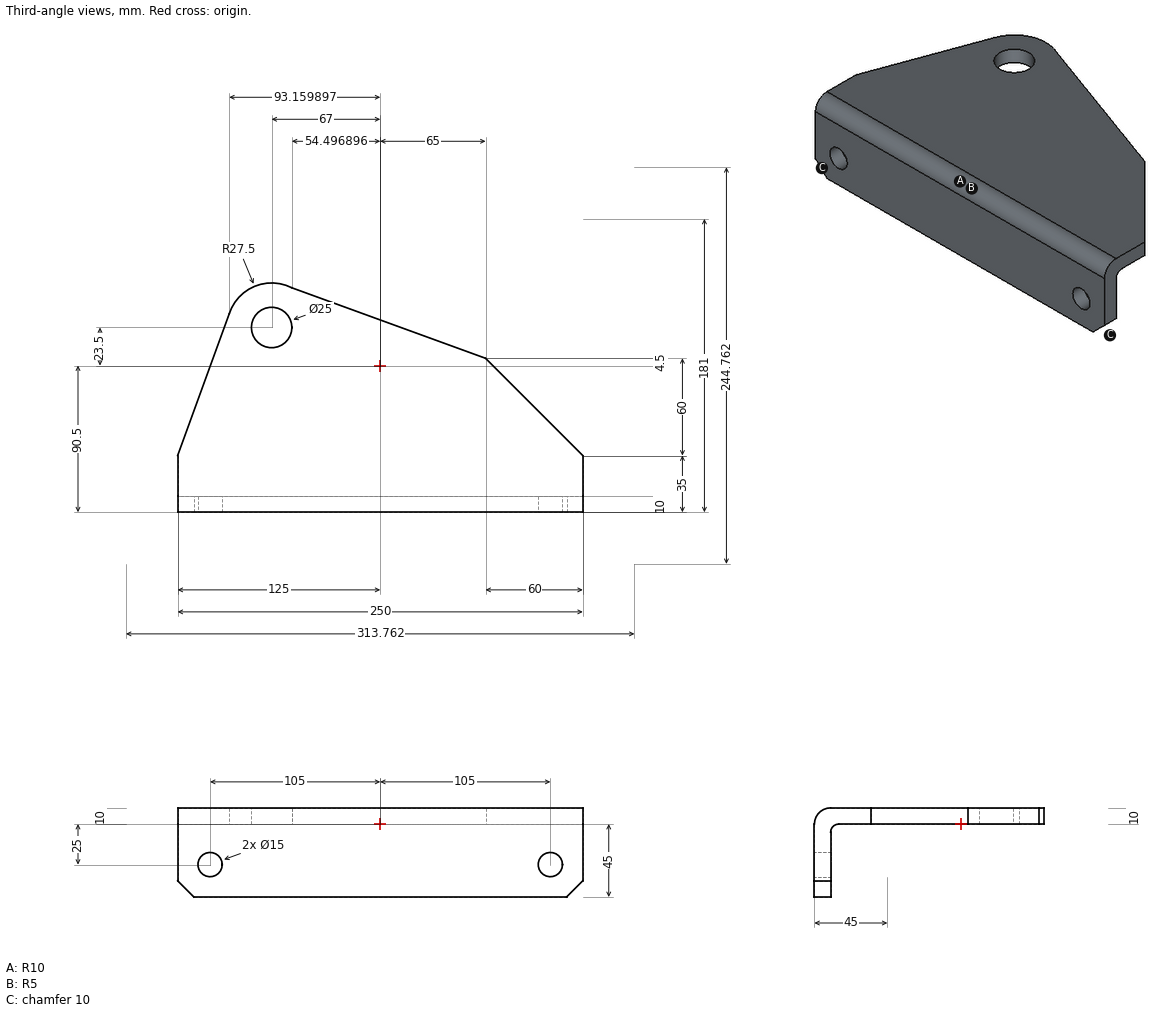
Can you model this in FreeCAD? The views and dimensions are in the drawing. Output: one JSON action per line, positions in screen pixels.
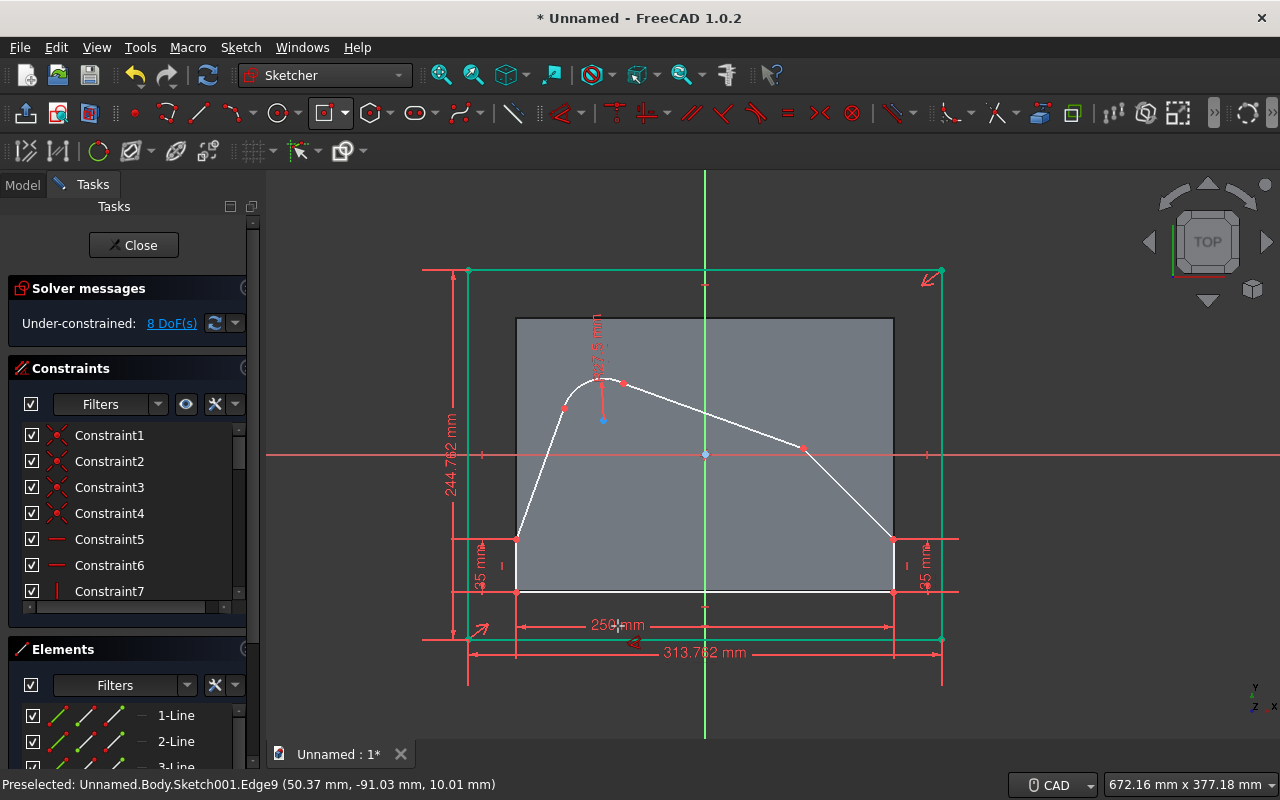
{"action": "left_click", "coordinate": [803, 449]}
{"action": "left_click", "coordinate": [754, 415]}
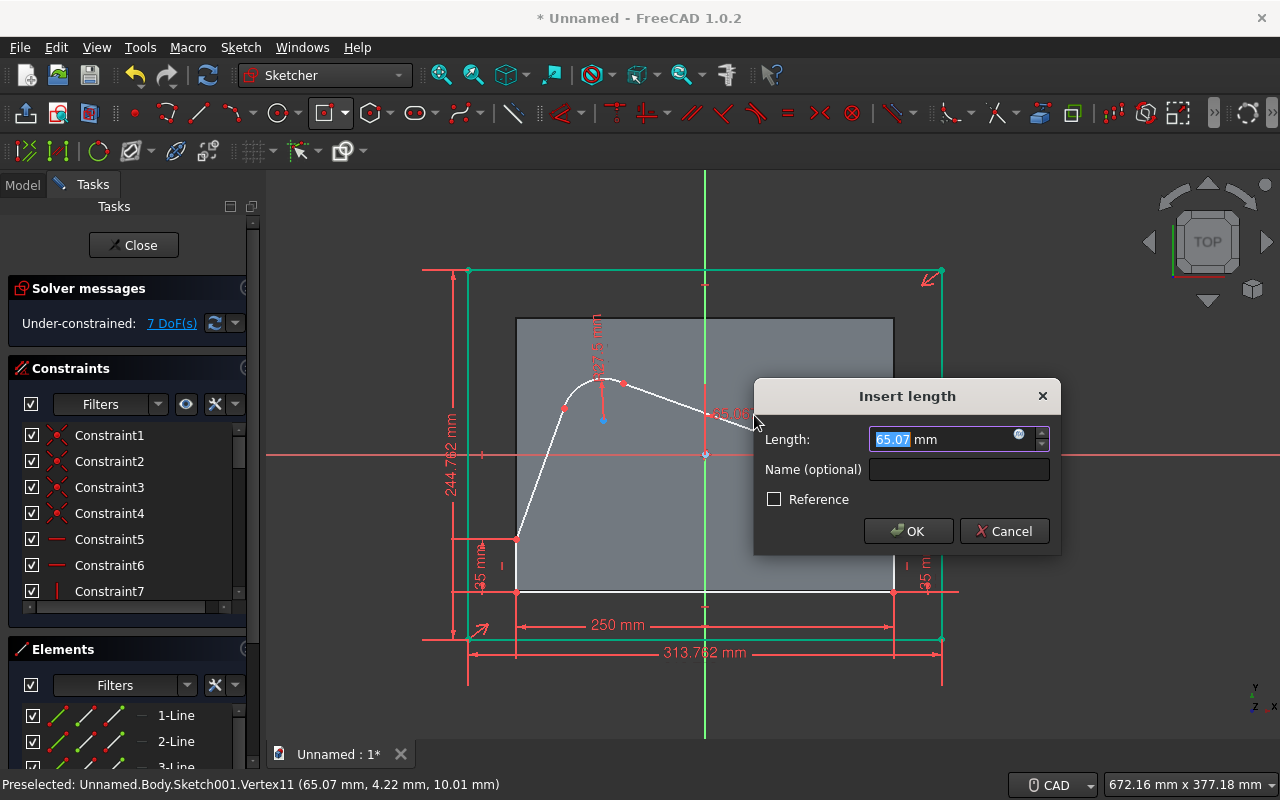
{"action": "type", "text": "65"}
{"action": "key", "text": "Return"}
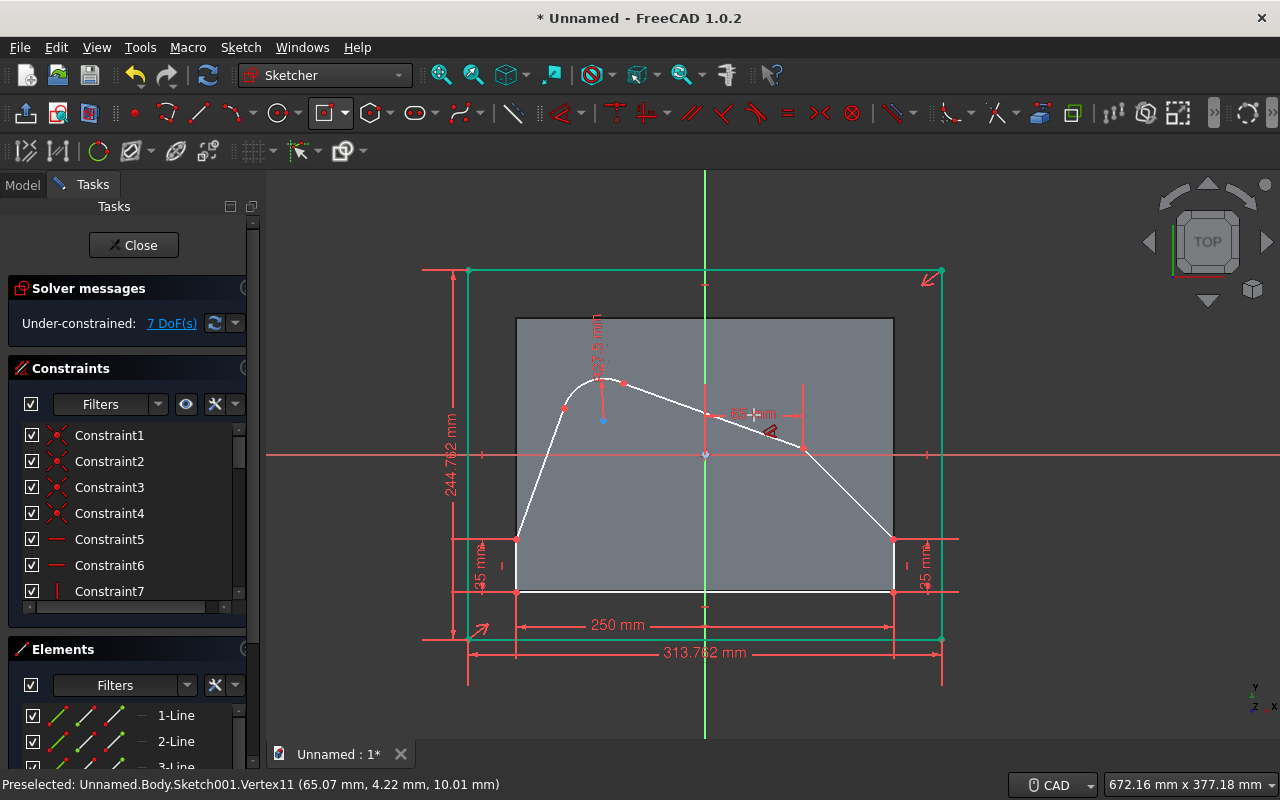
{"action": "left_click", "coordinate": [830, 476]}
{"action": "left_click", "coordinate": [848, 573]}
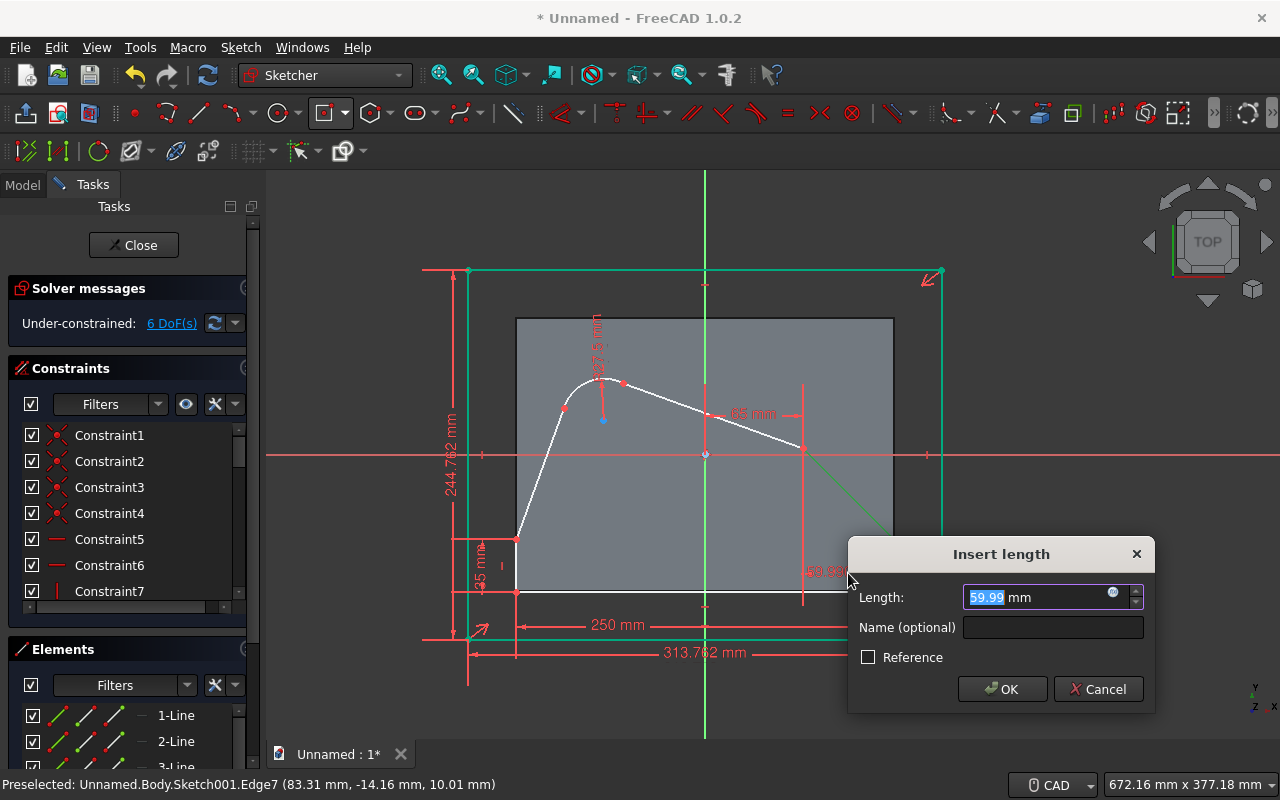
{"action": "type", "text": "60"}
{"action": "key", "text": "Return"}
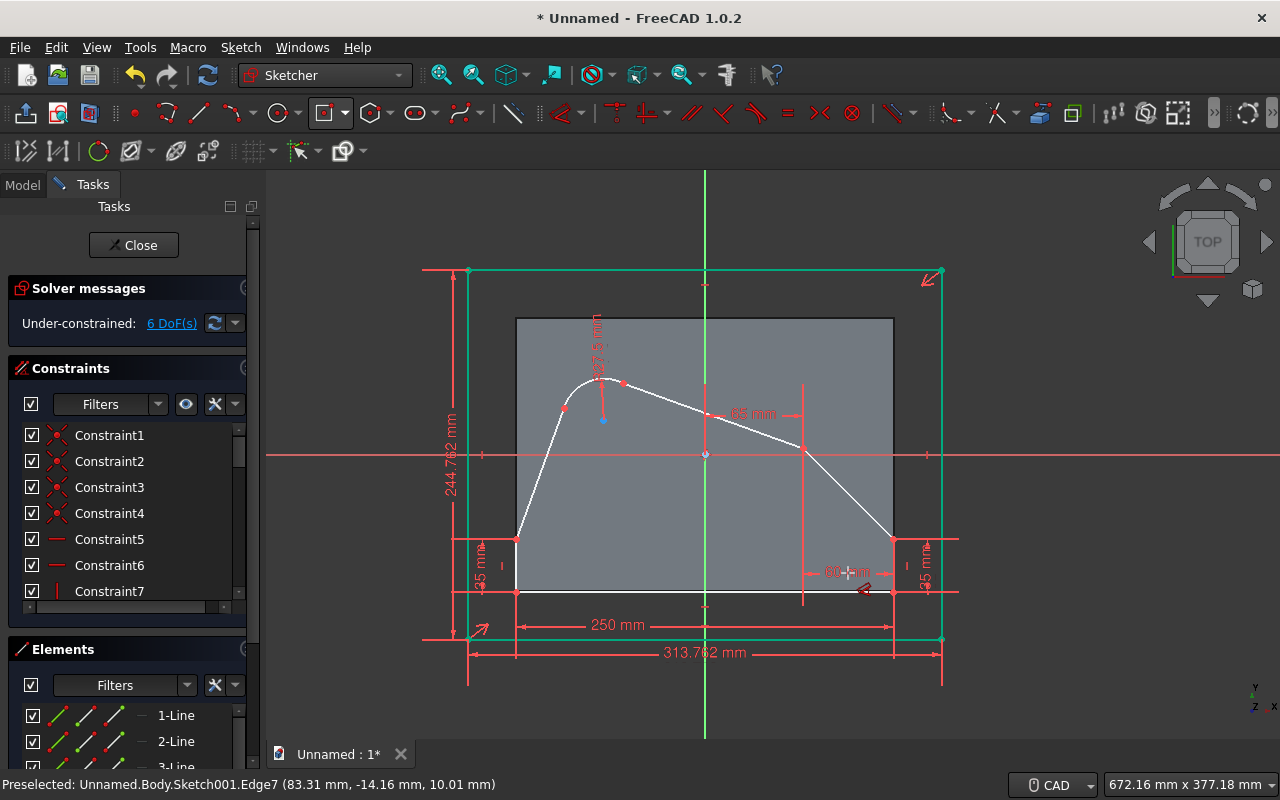
{"action": "left_click", "coordinate": [830, 476]}
{"action": "left_click", "coordinate": [928, 494]}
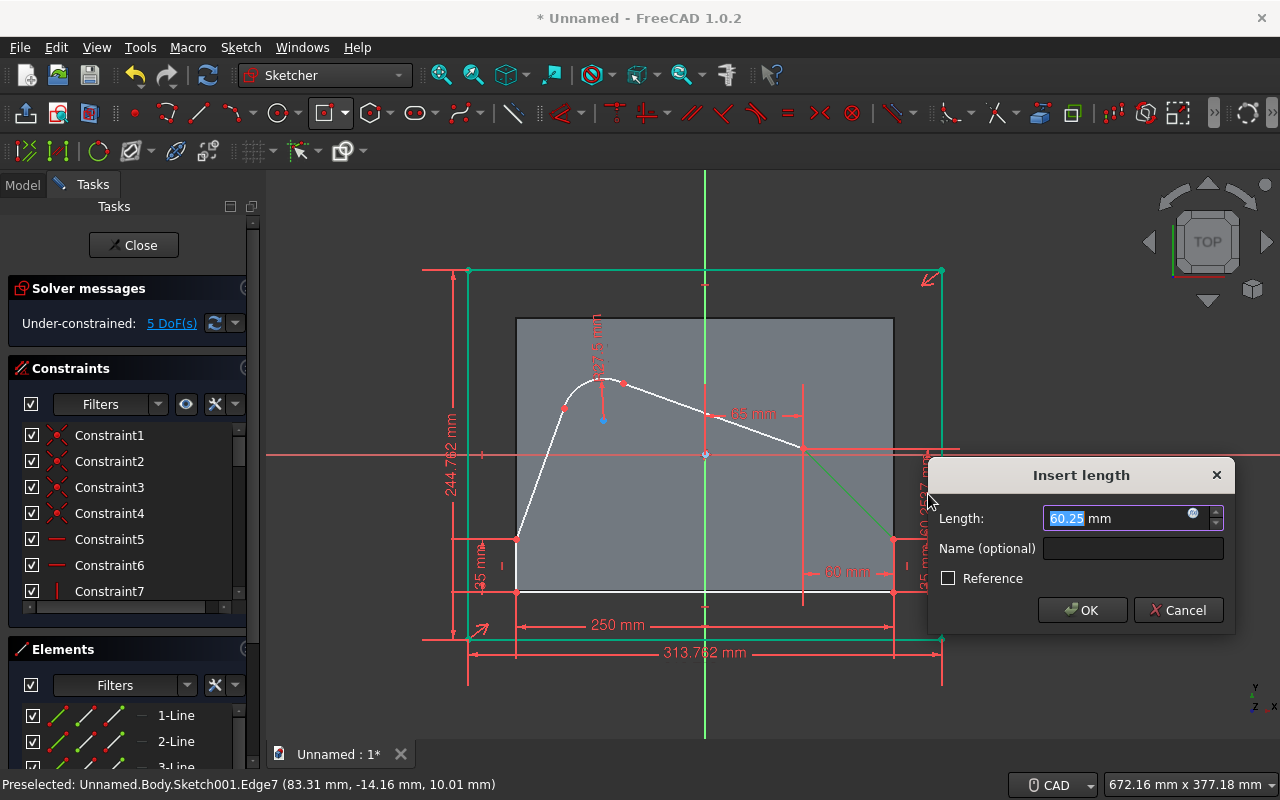
{"action": "type", "text": "60"}
{"action": "key", "text": "Return"}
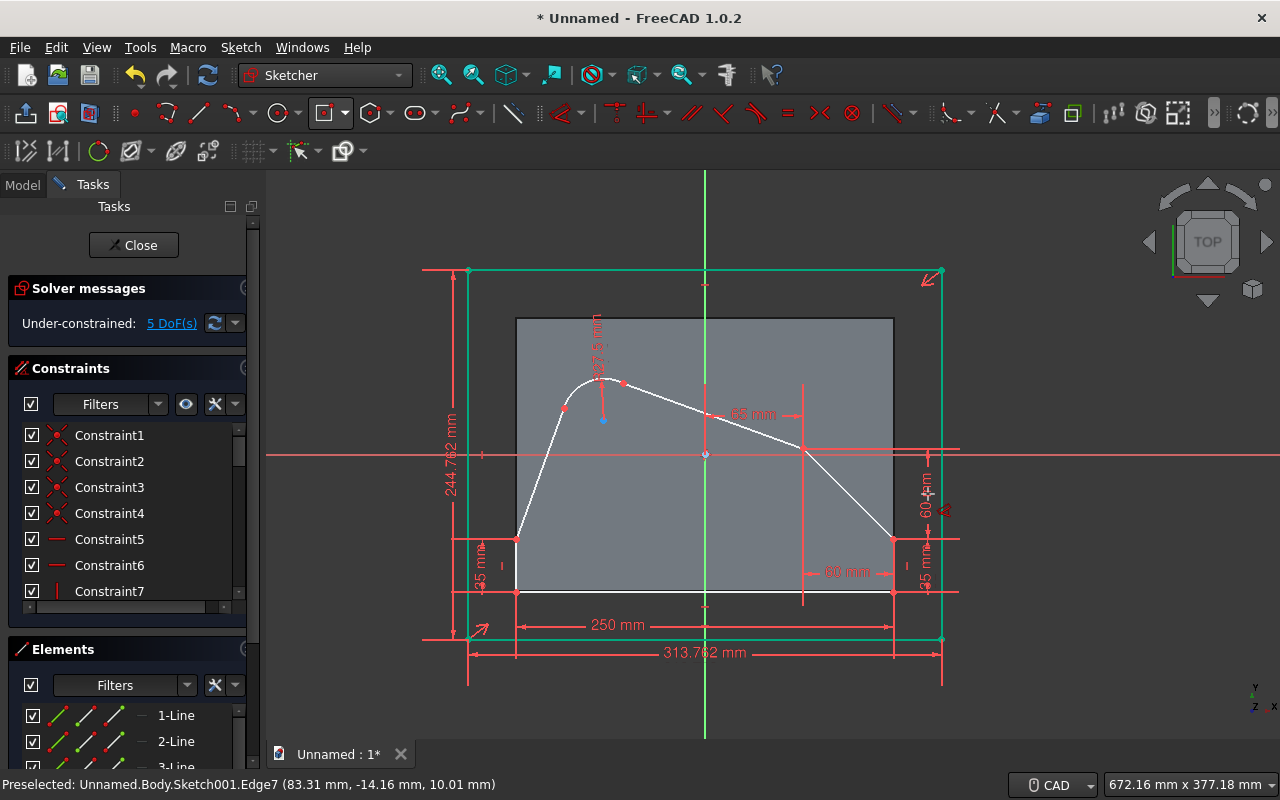
{"action": "left_click", "coordinate": [604, 420]}
{"action": "left_click", "coordinate": [678, 386]}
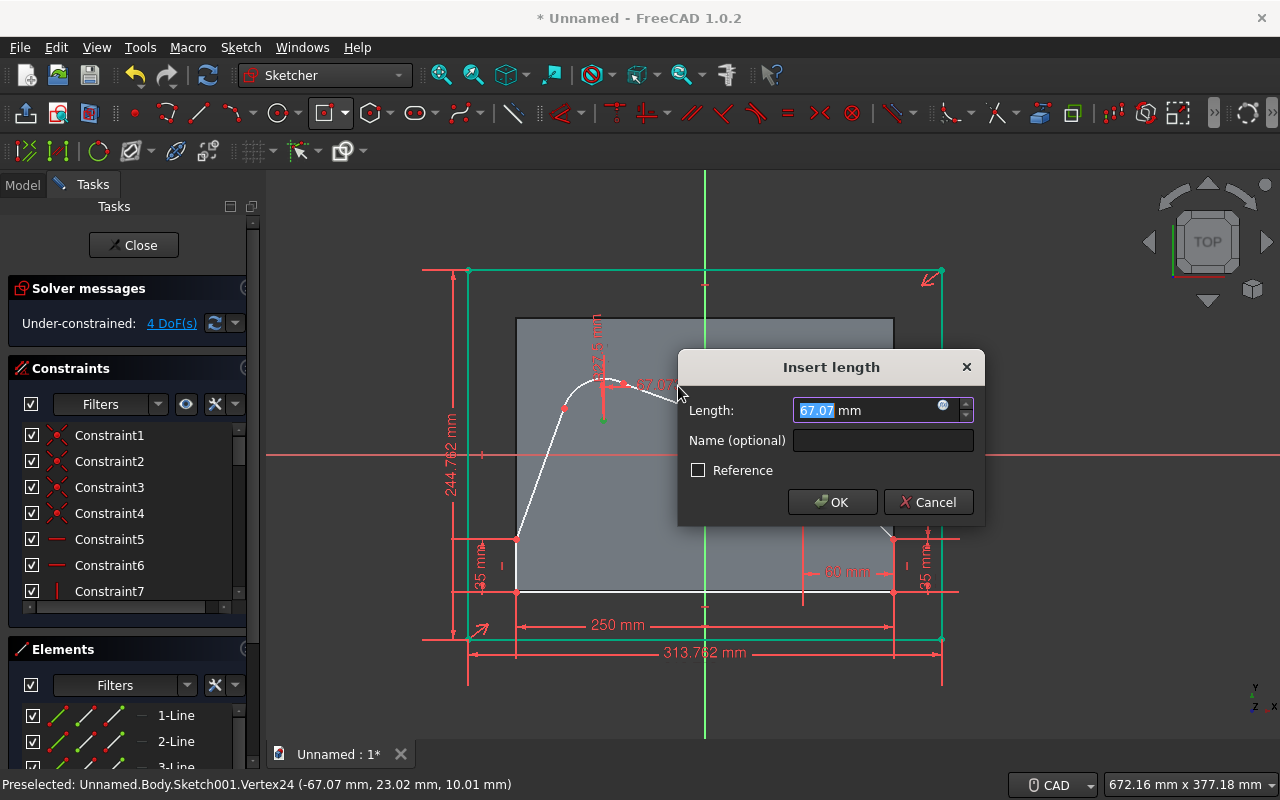
{"action": "type", "text": "67"}
{"action": "key", "text": "Return"}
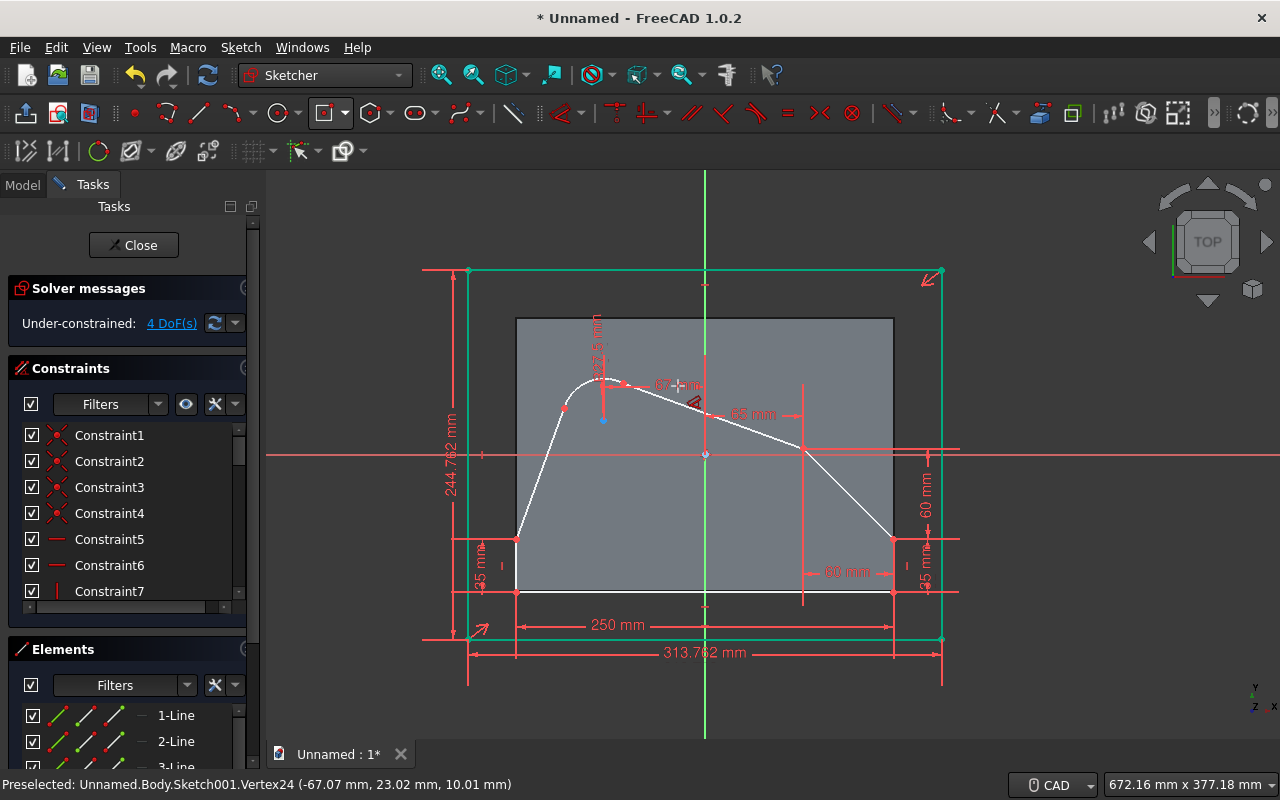
{"action": "scroll", "coordinate": [803, 449], "scroll_direction": "up", "scroll_amount": 9}